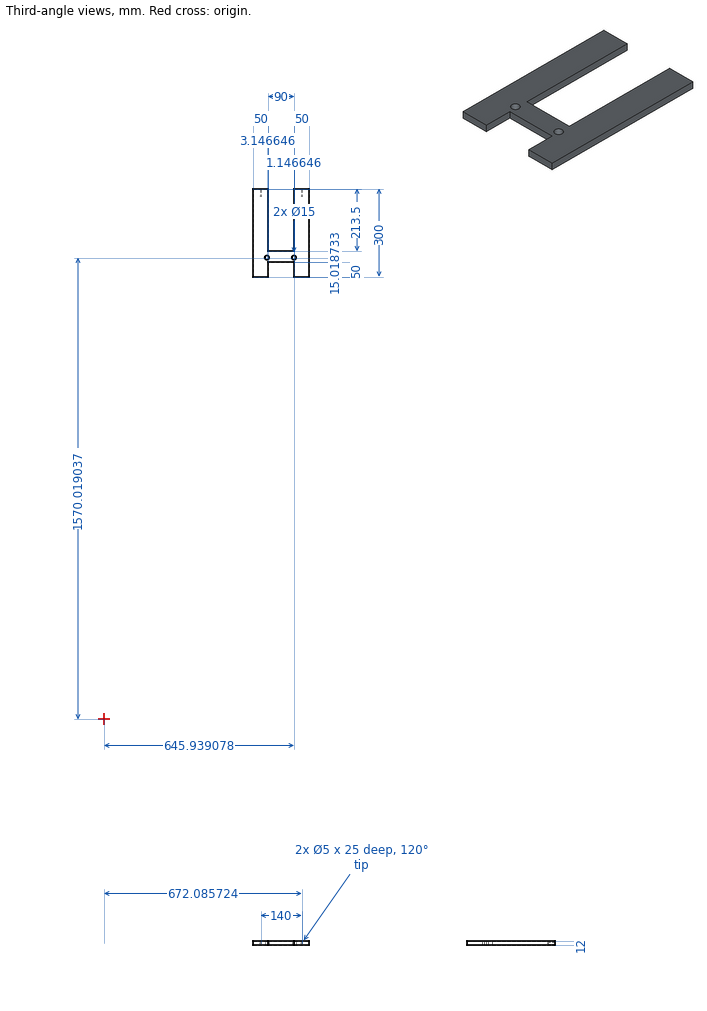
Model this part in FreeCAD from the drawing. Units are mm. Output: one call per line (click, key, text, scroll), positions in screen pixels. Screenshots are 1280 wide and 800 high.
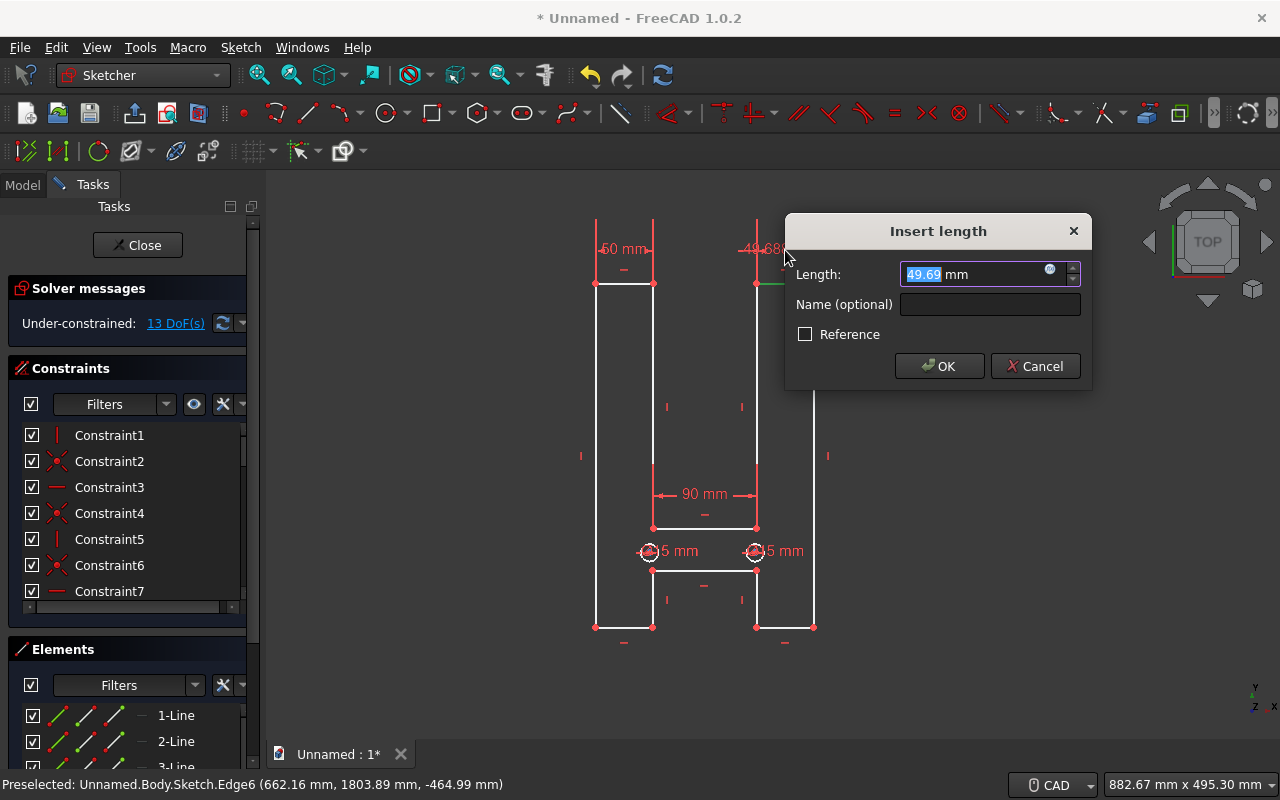
text(50)
key(Return)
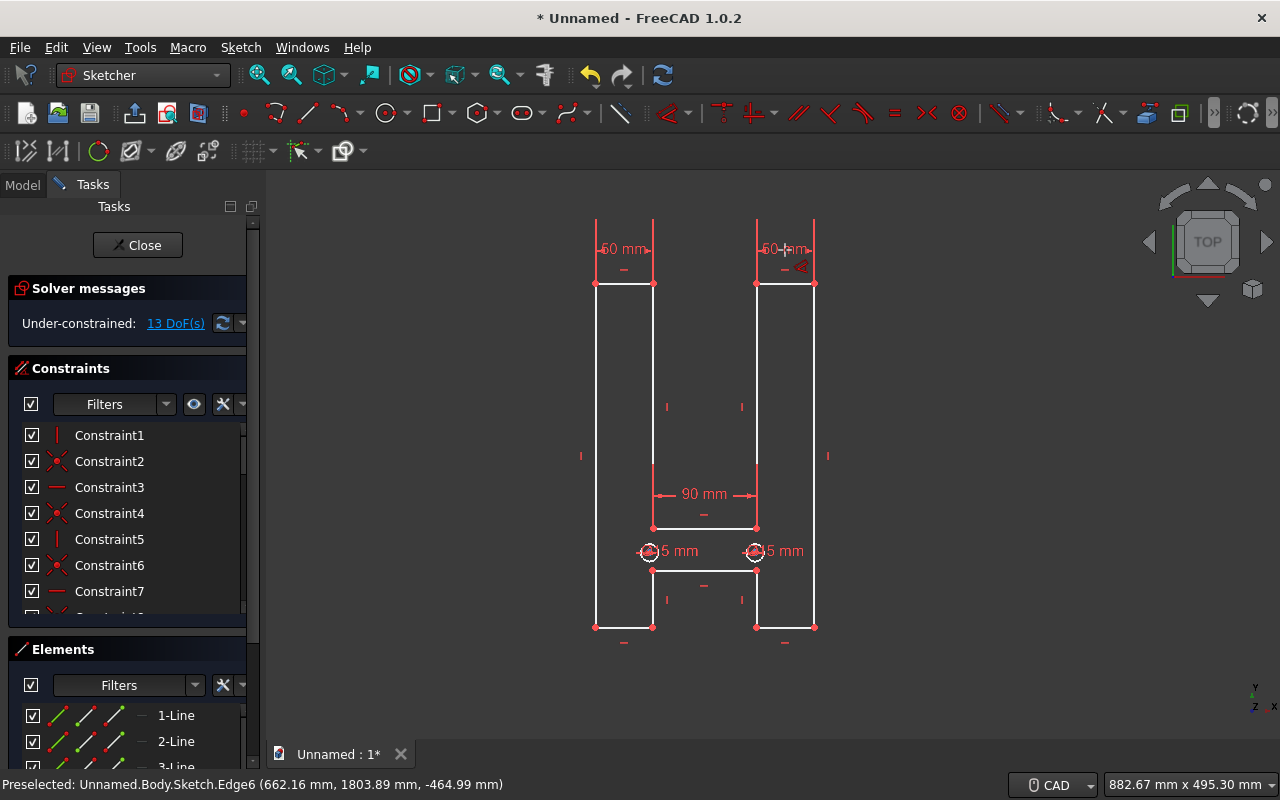
click(797, 628)
click(785, 662)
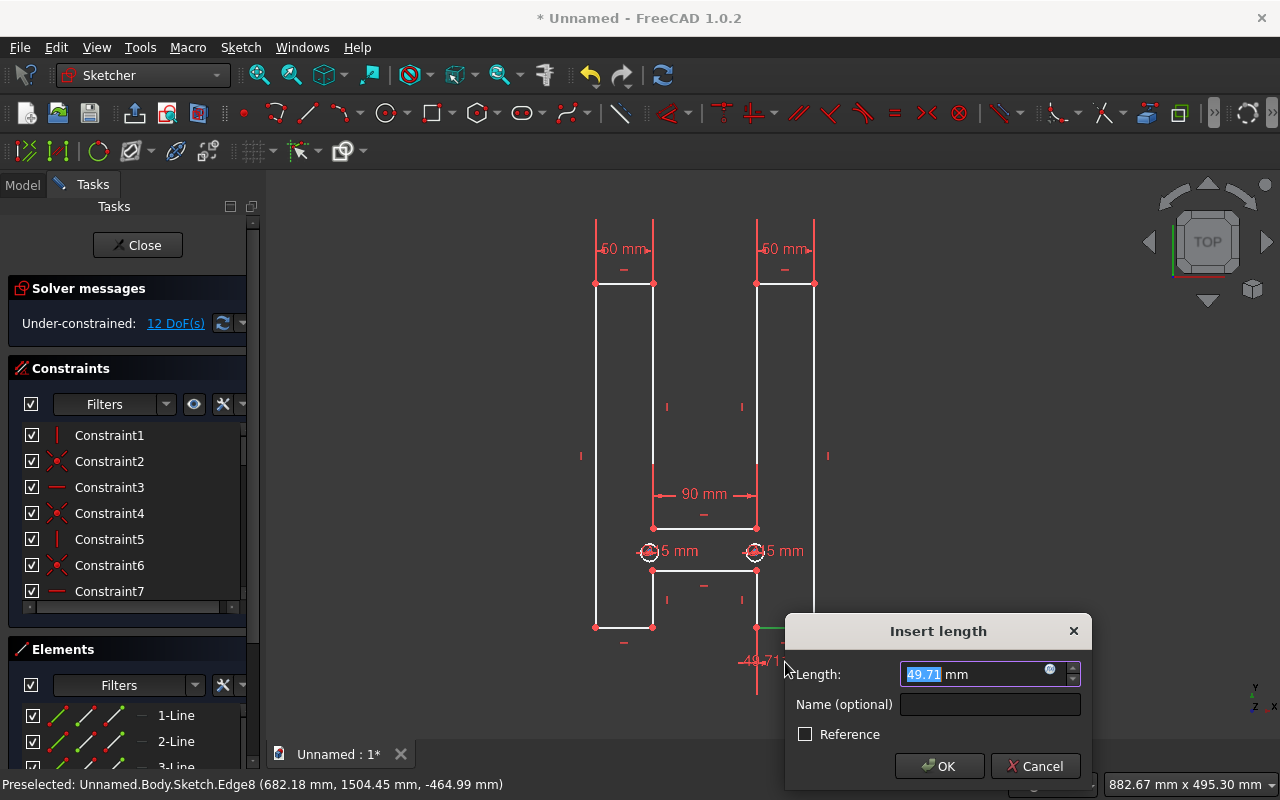
text(50)
key(Return)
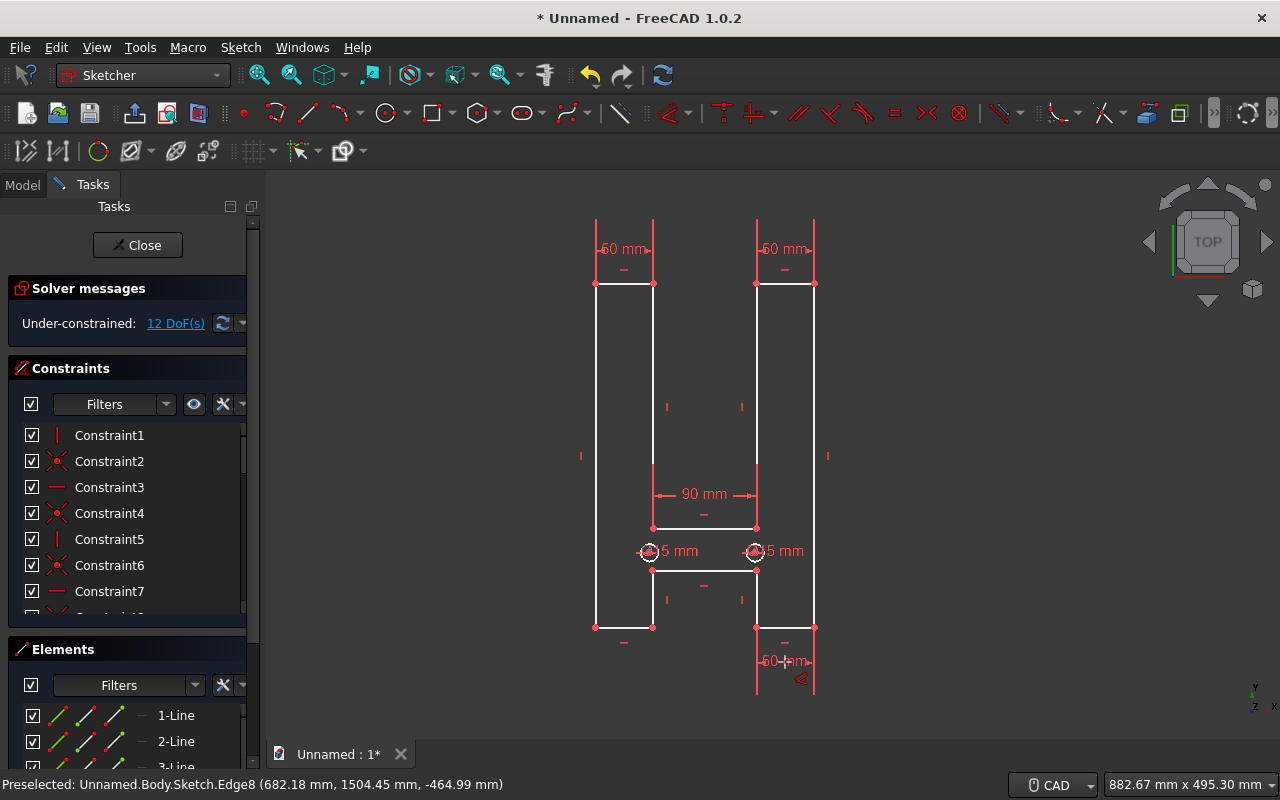
click(757, 611)
click(791, 599)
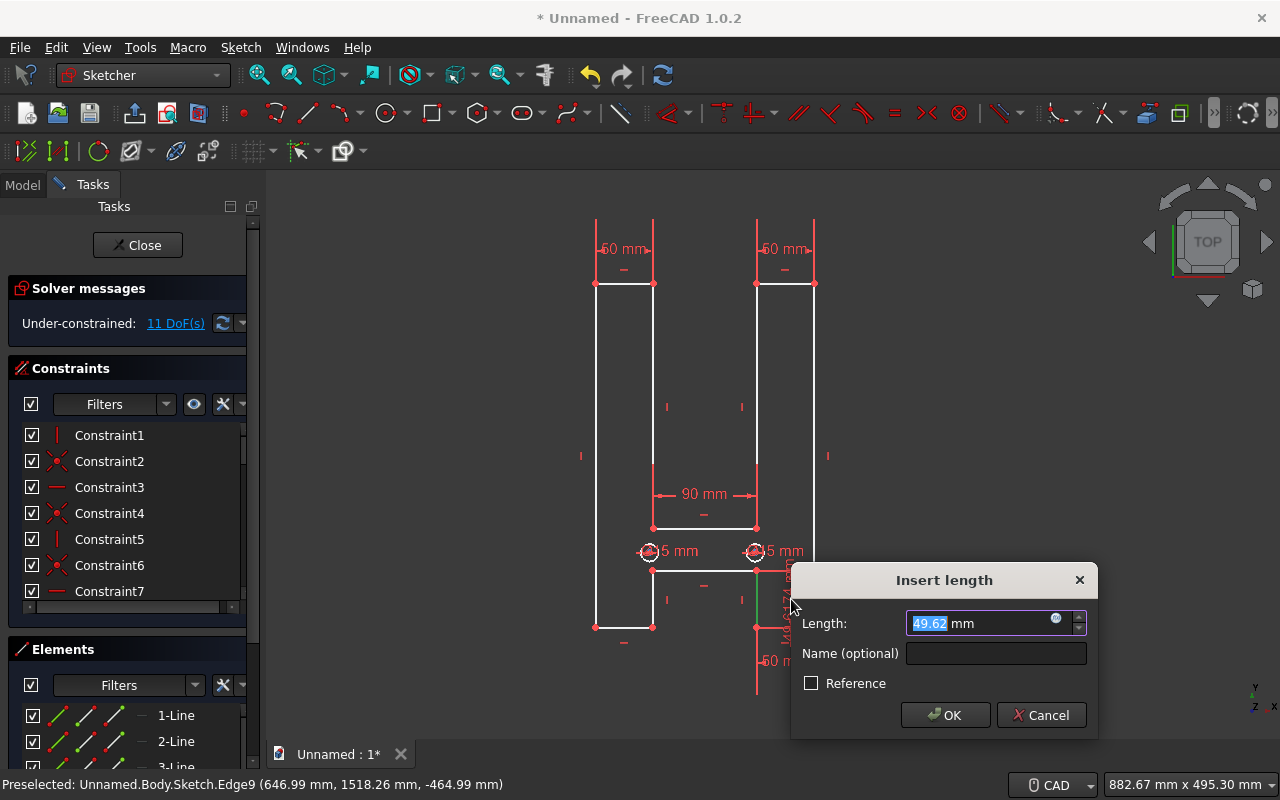
text(50)
key(Return)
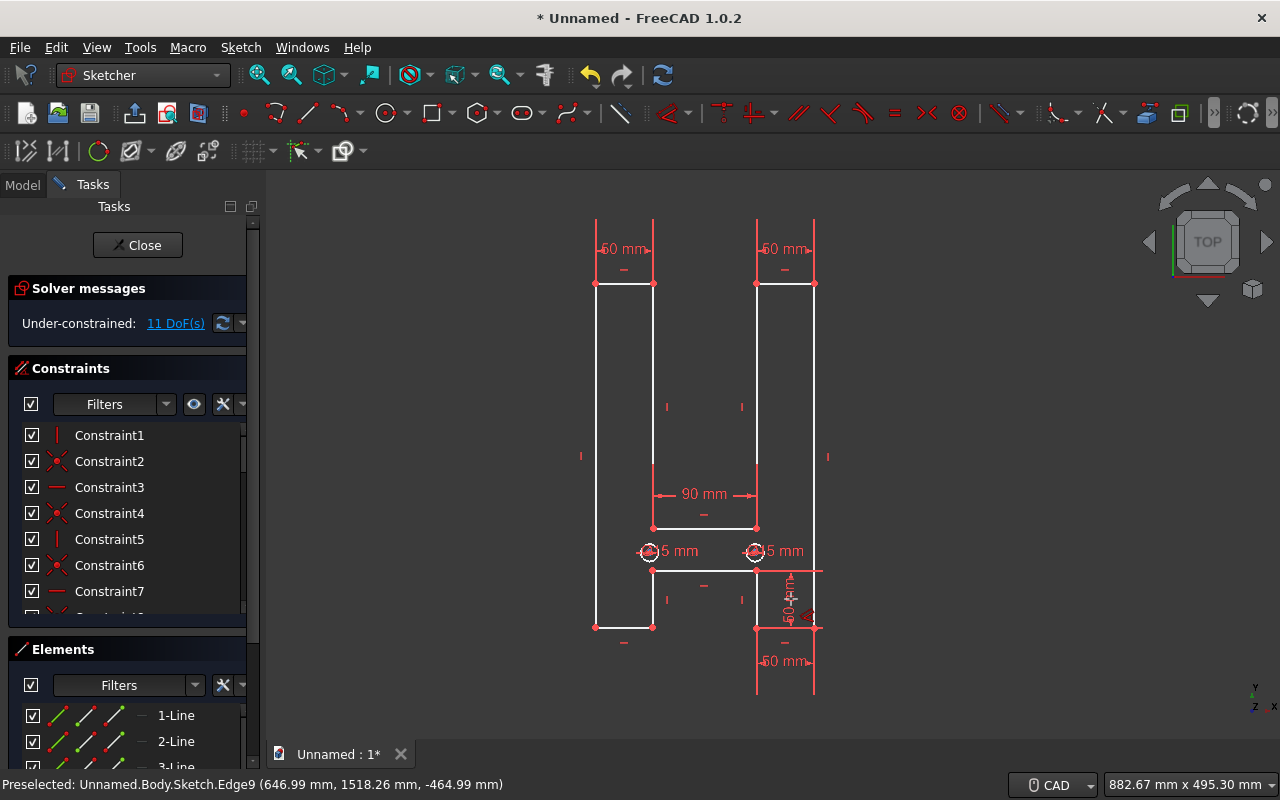
click(725, 571)
click(705, 605)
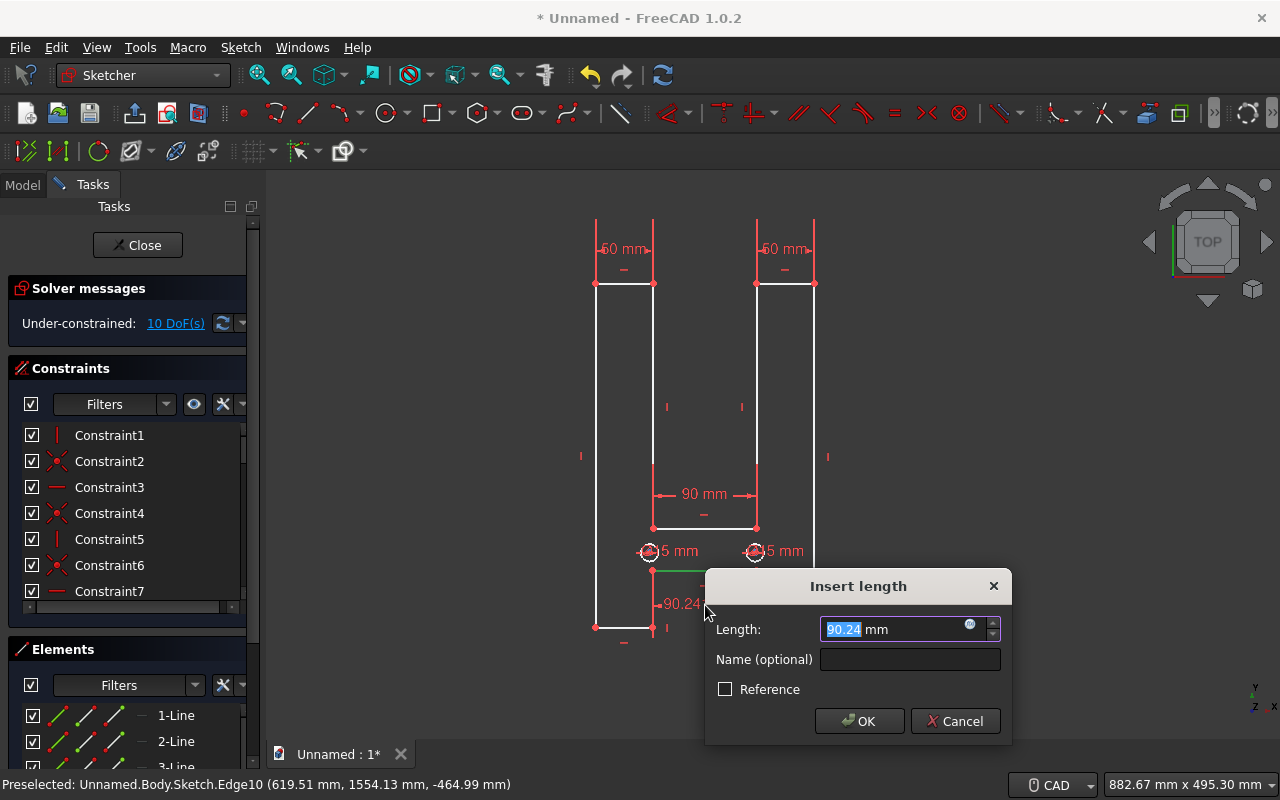
text(90)
key(Return)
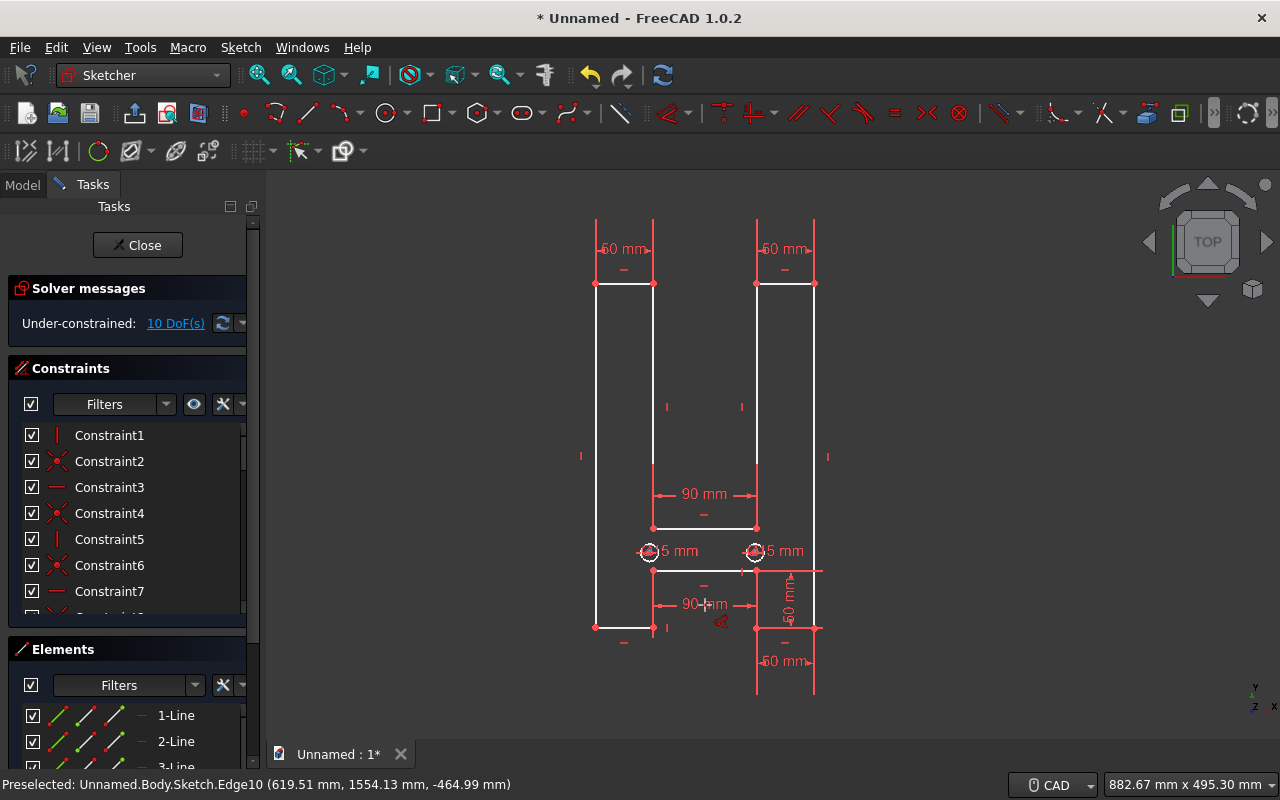
click(653, 588)
click(619, 599)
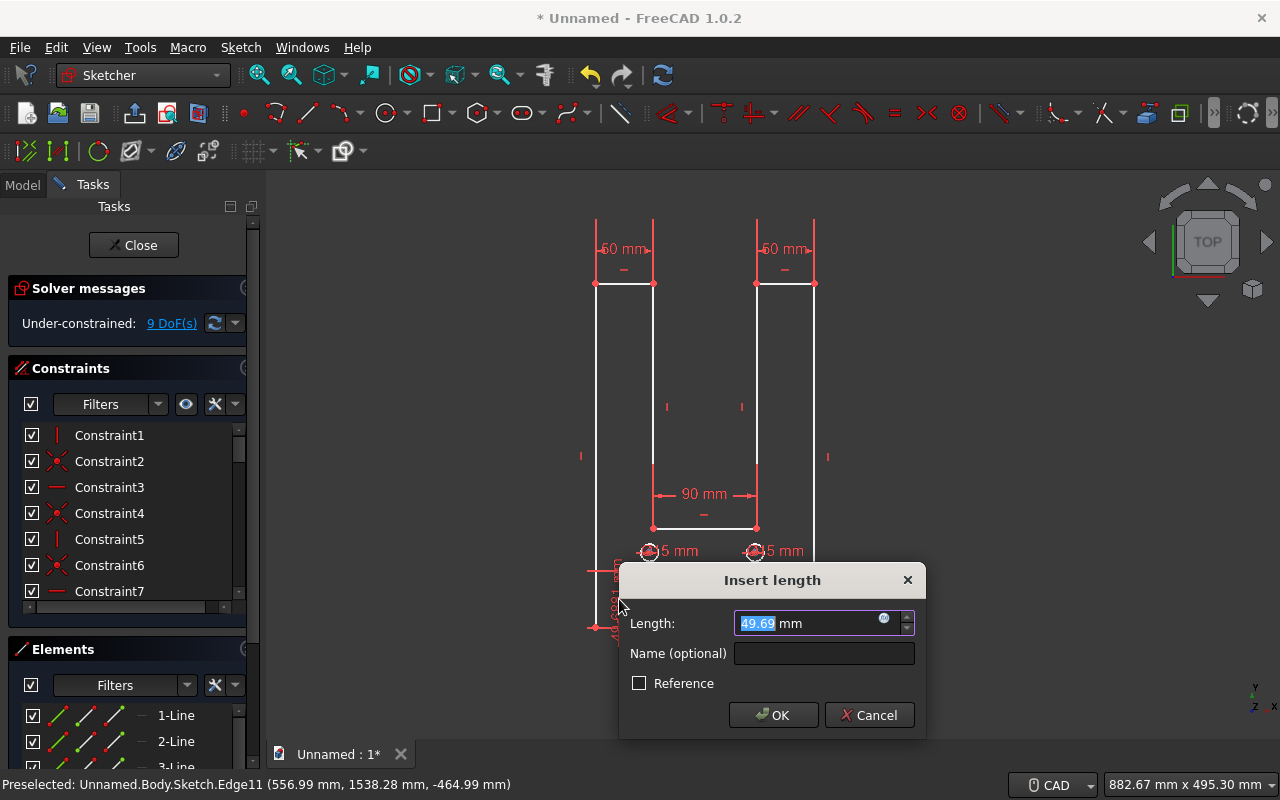
text(50)
key(Return)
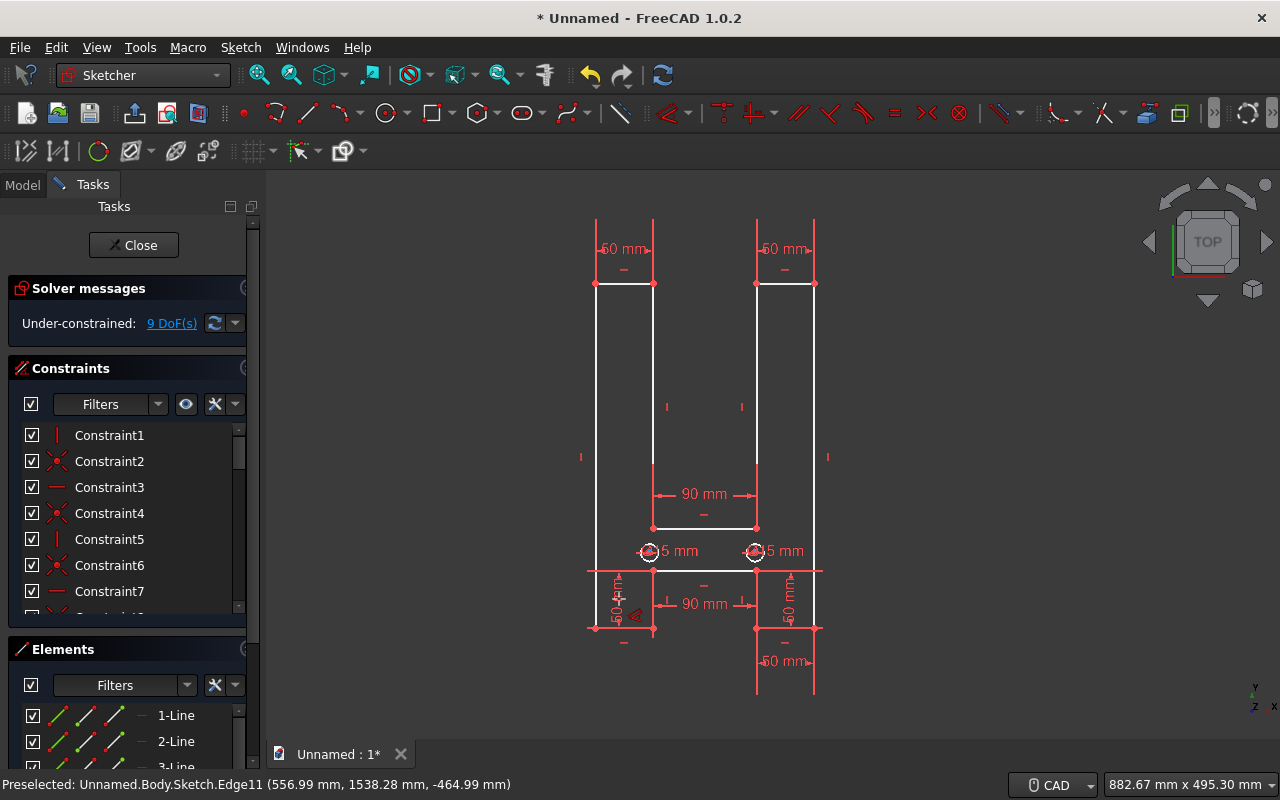
click(596, 525)
click(562, 456)